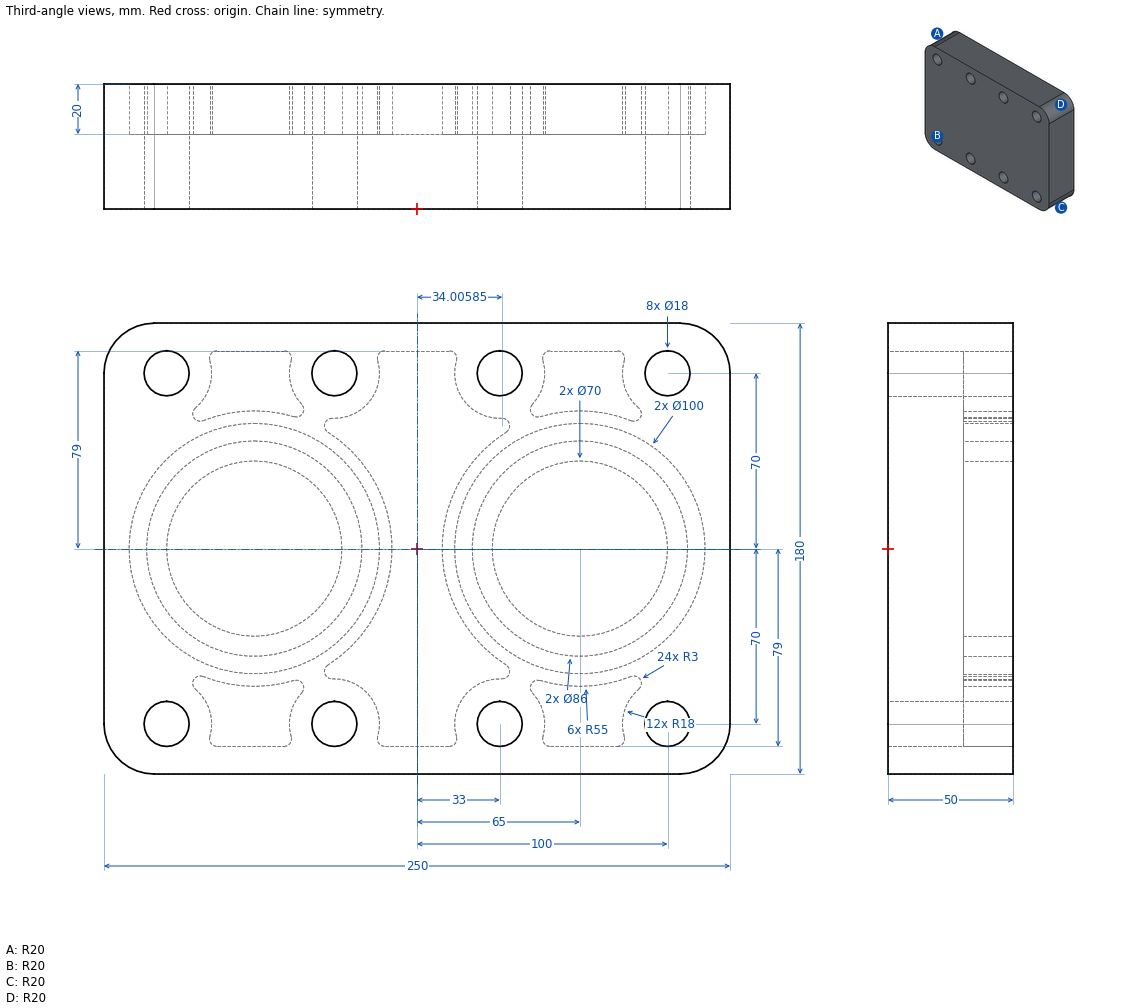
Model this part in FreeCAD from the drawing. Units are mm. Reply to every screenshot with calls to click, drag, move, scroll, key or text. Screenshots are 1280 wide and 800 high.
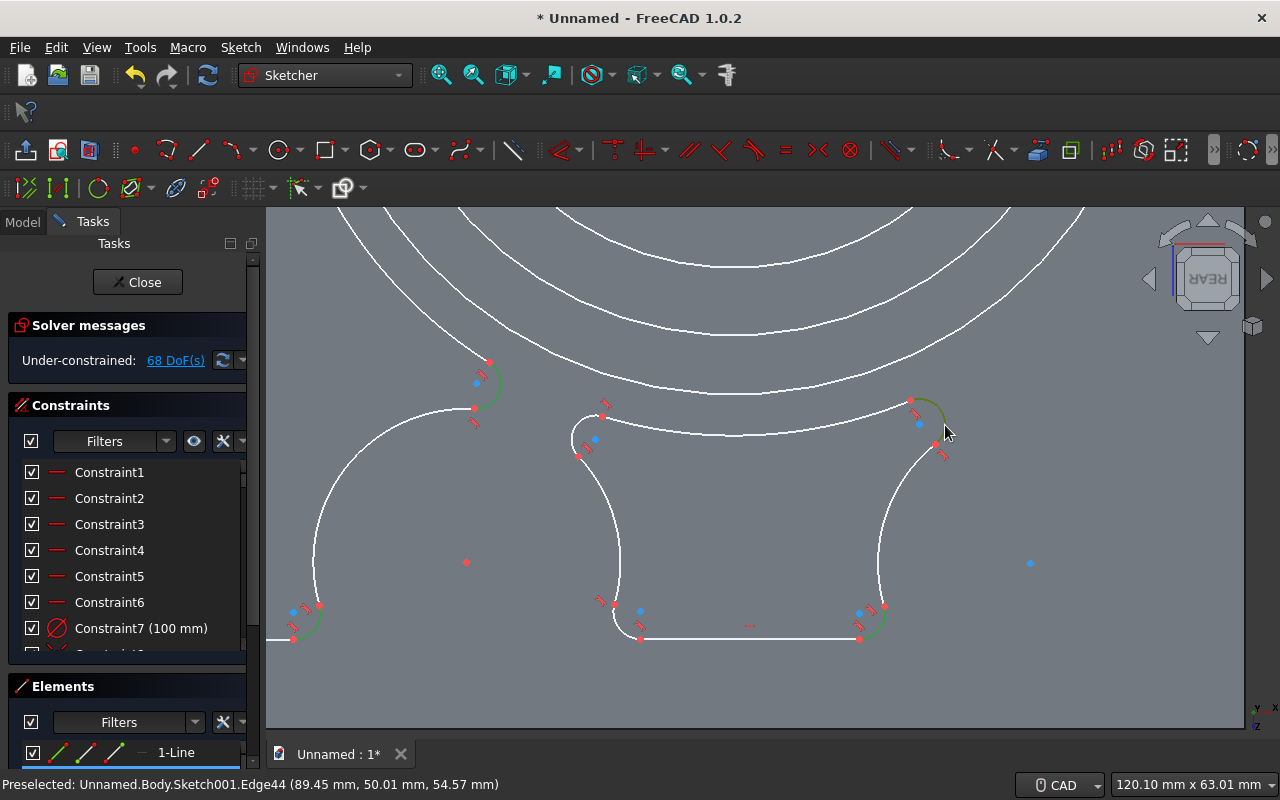
click(584, 418)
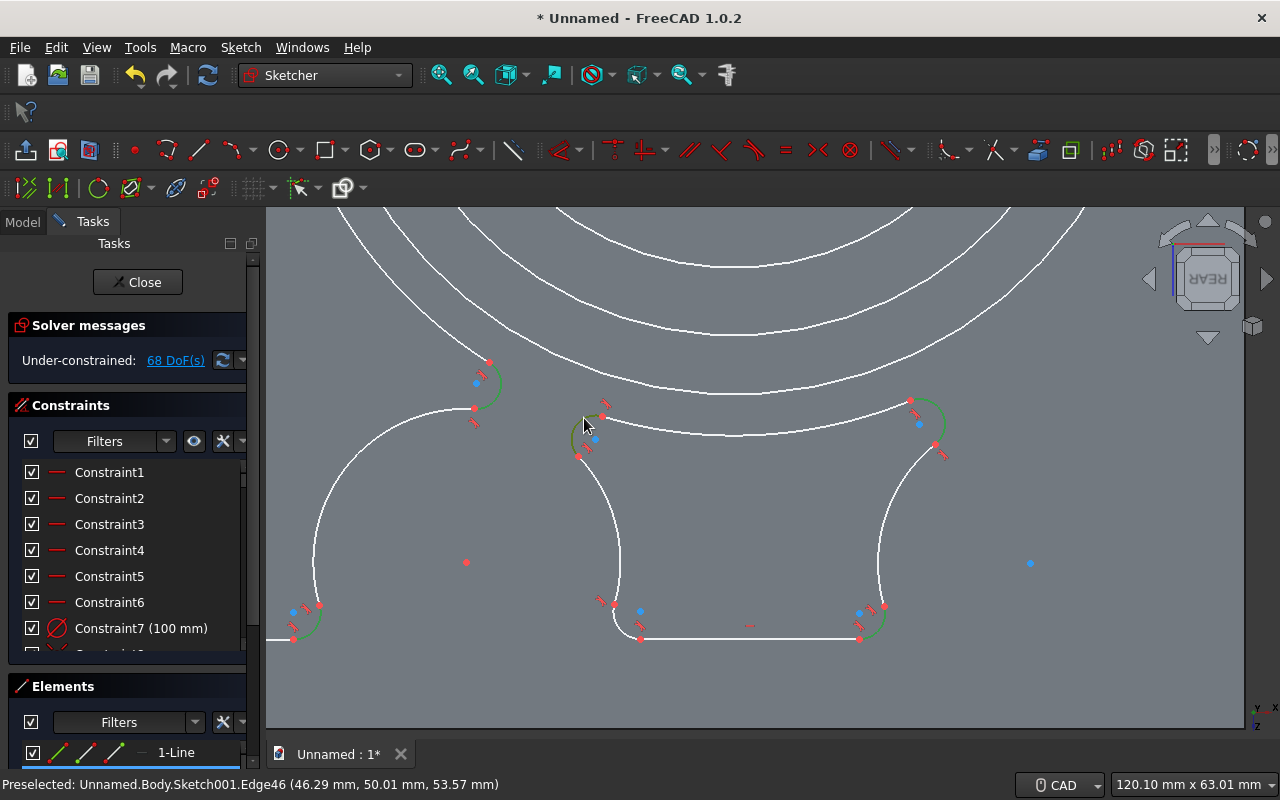
click(615, 619)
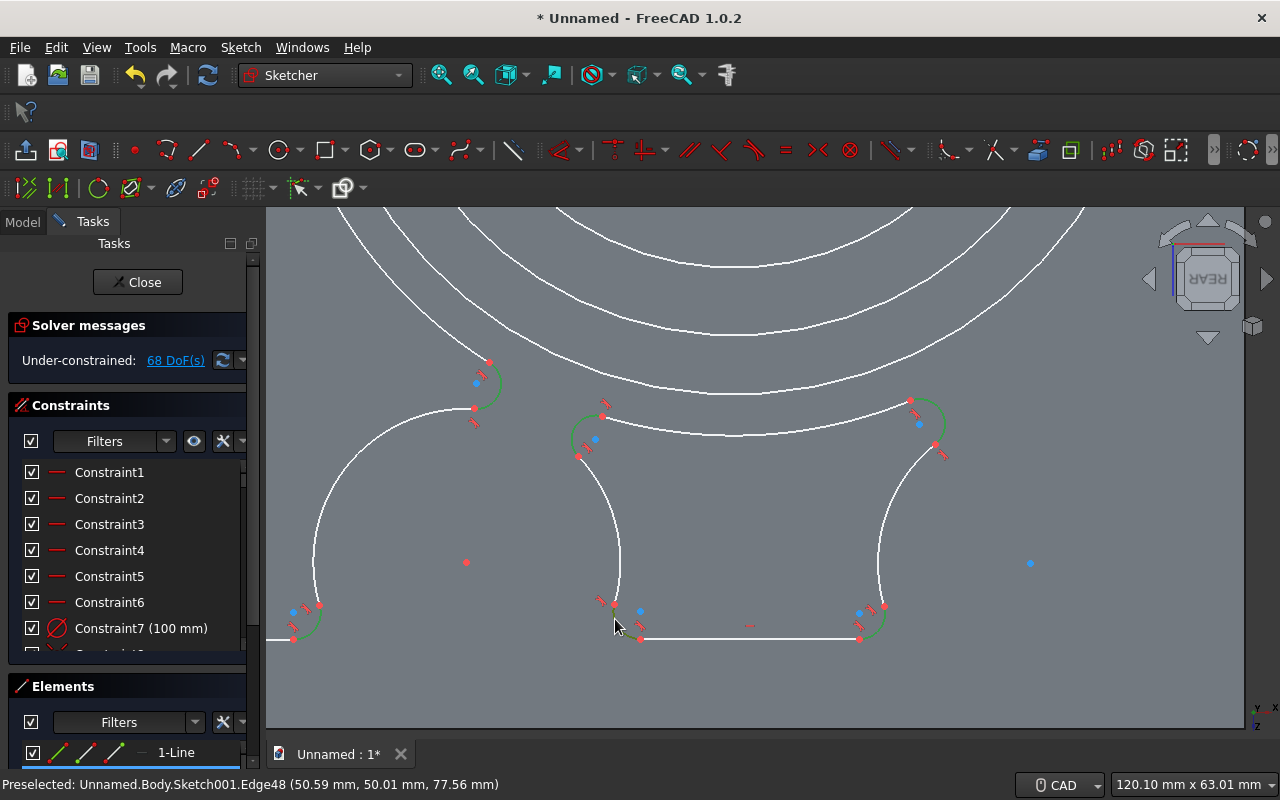
click(786, 150)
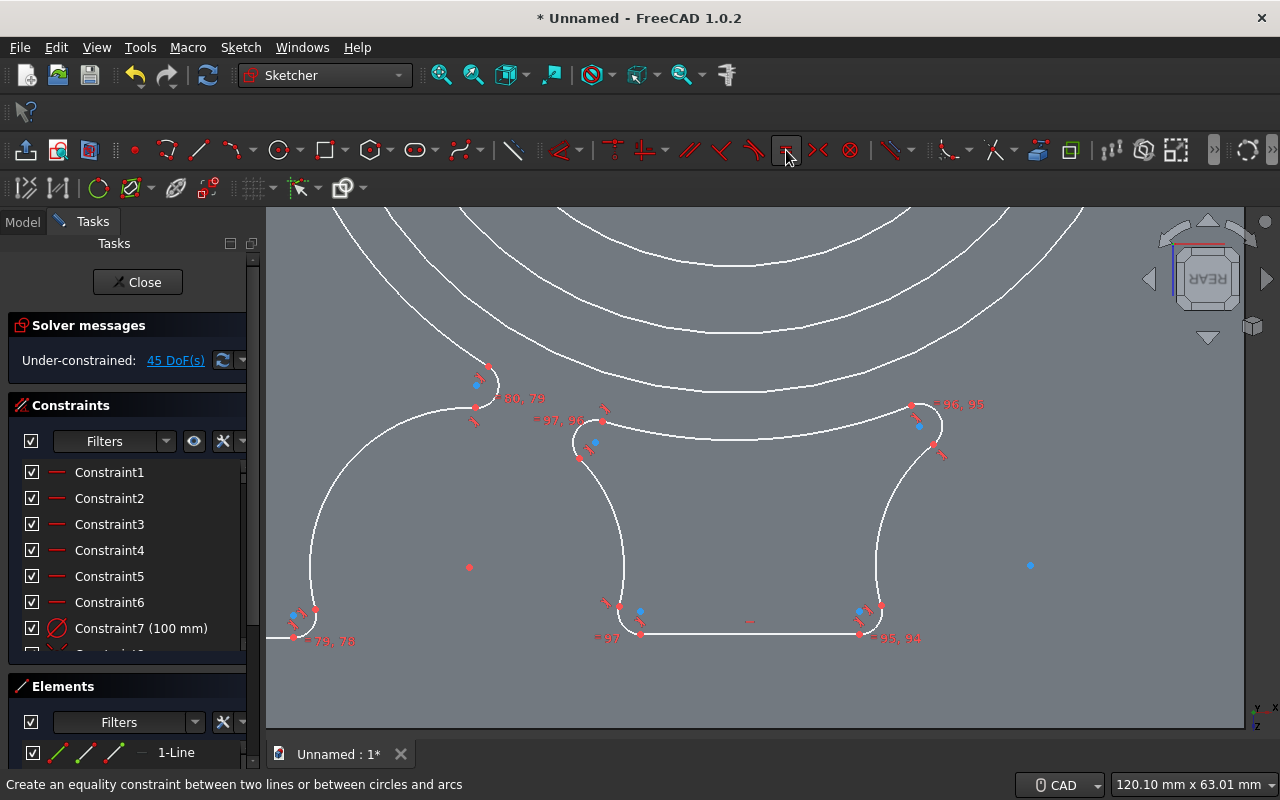
scroll(873, 638, down, 7)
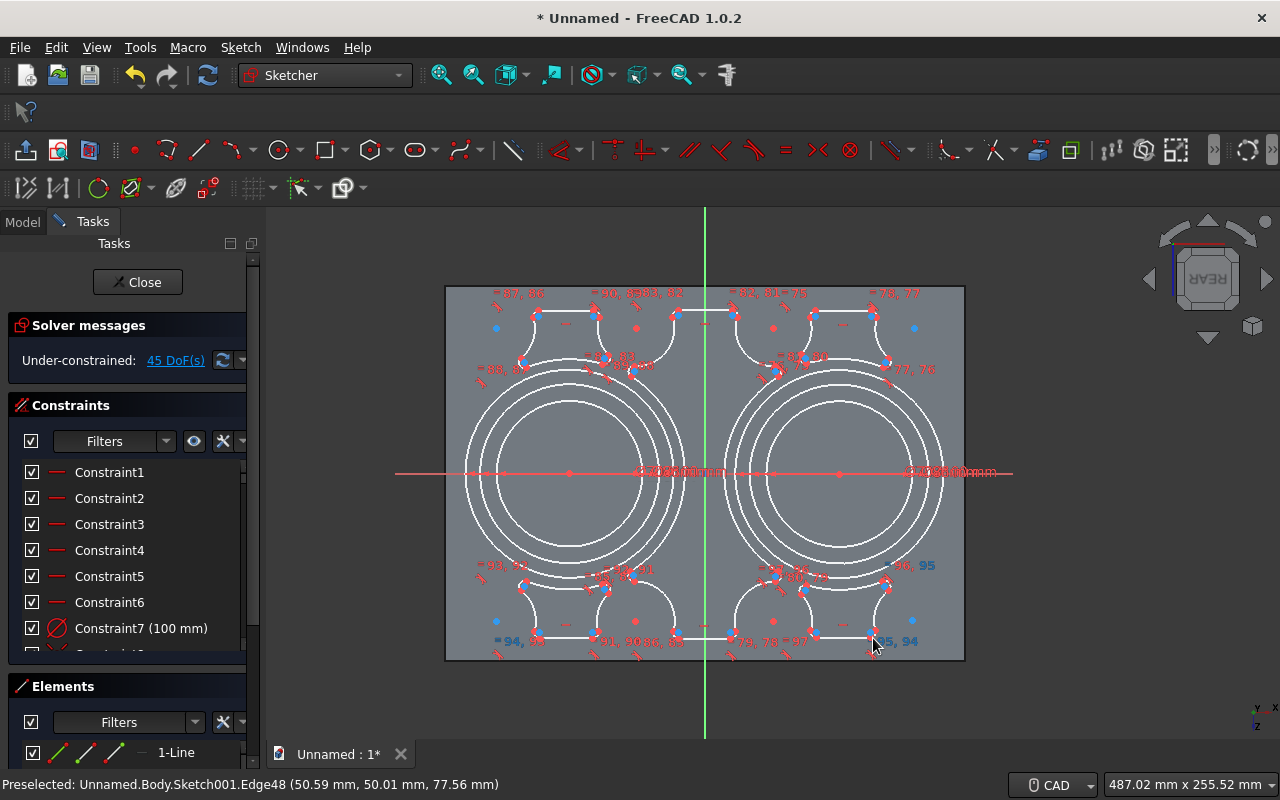
click(808, 345)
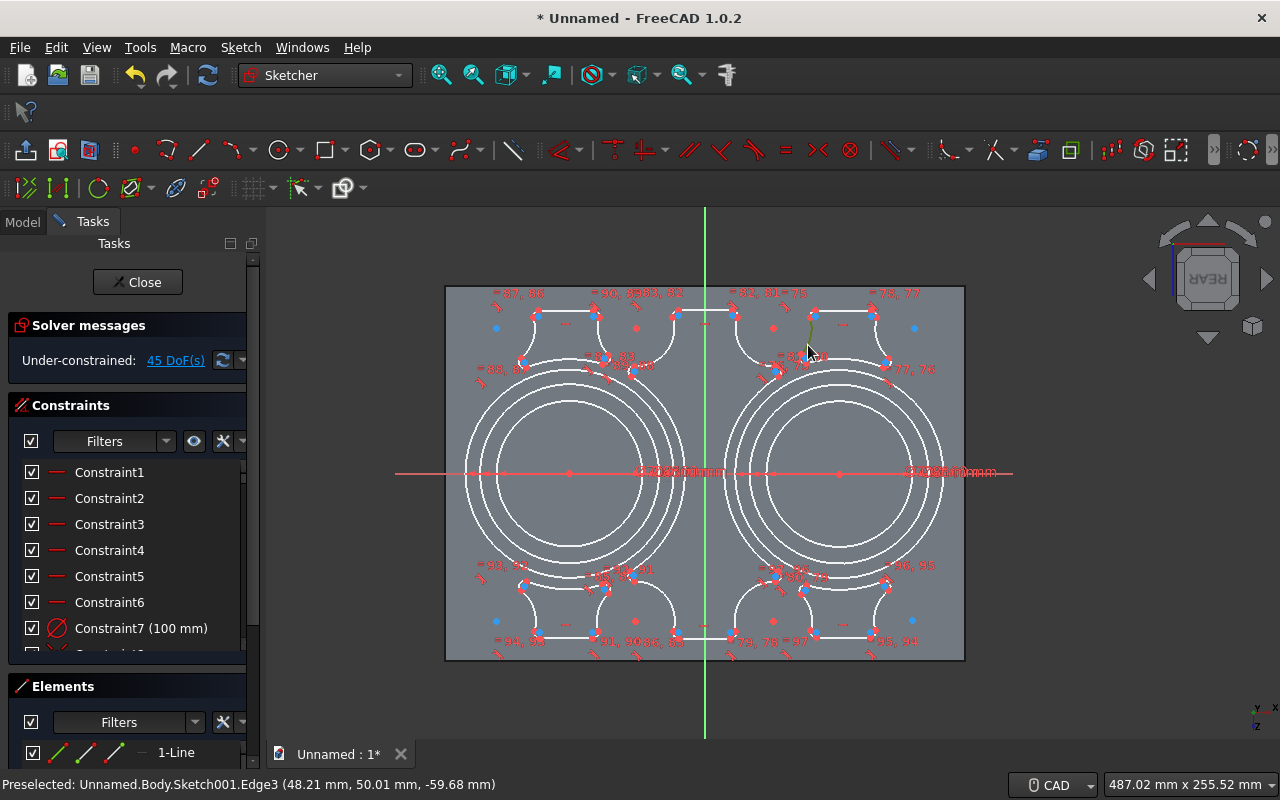
click(875, 331)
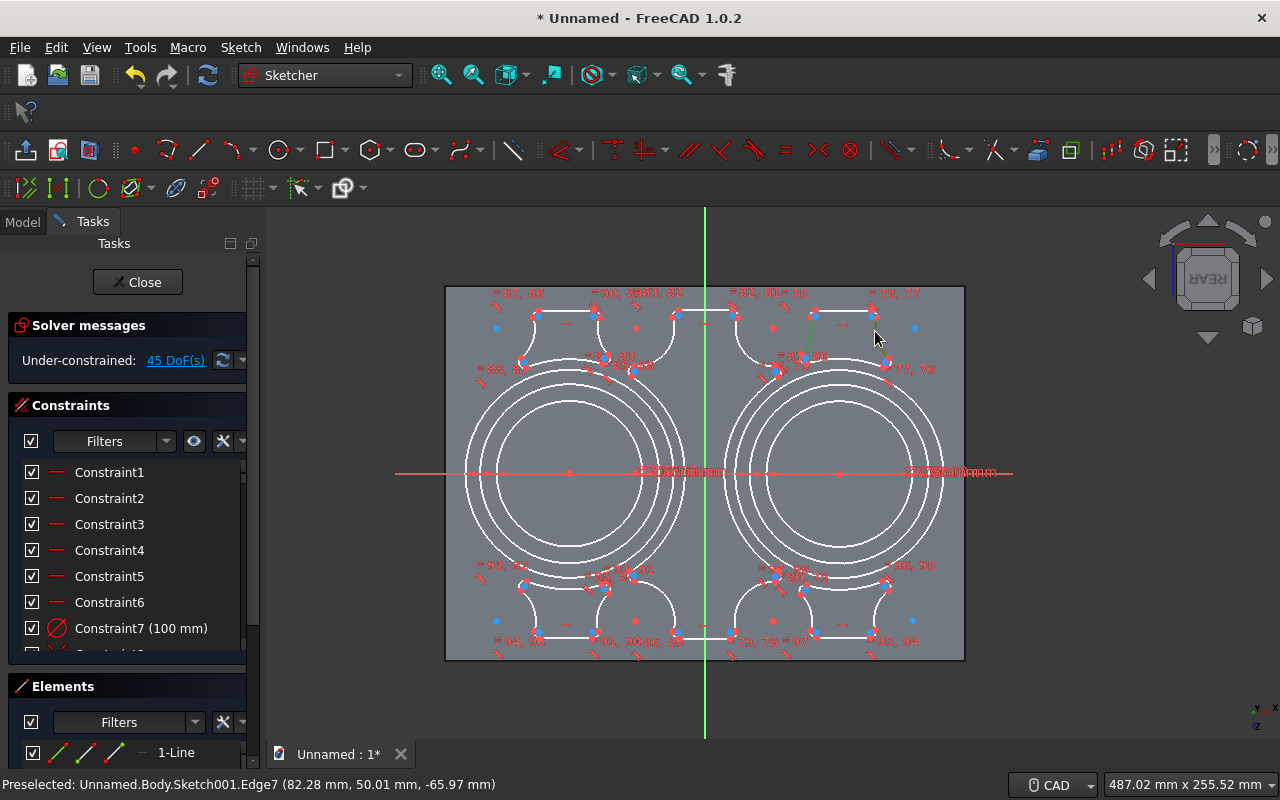
click(754, 587)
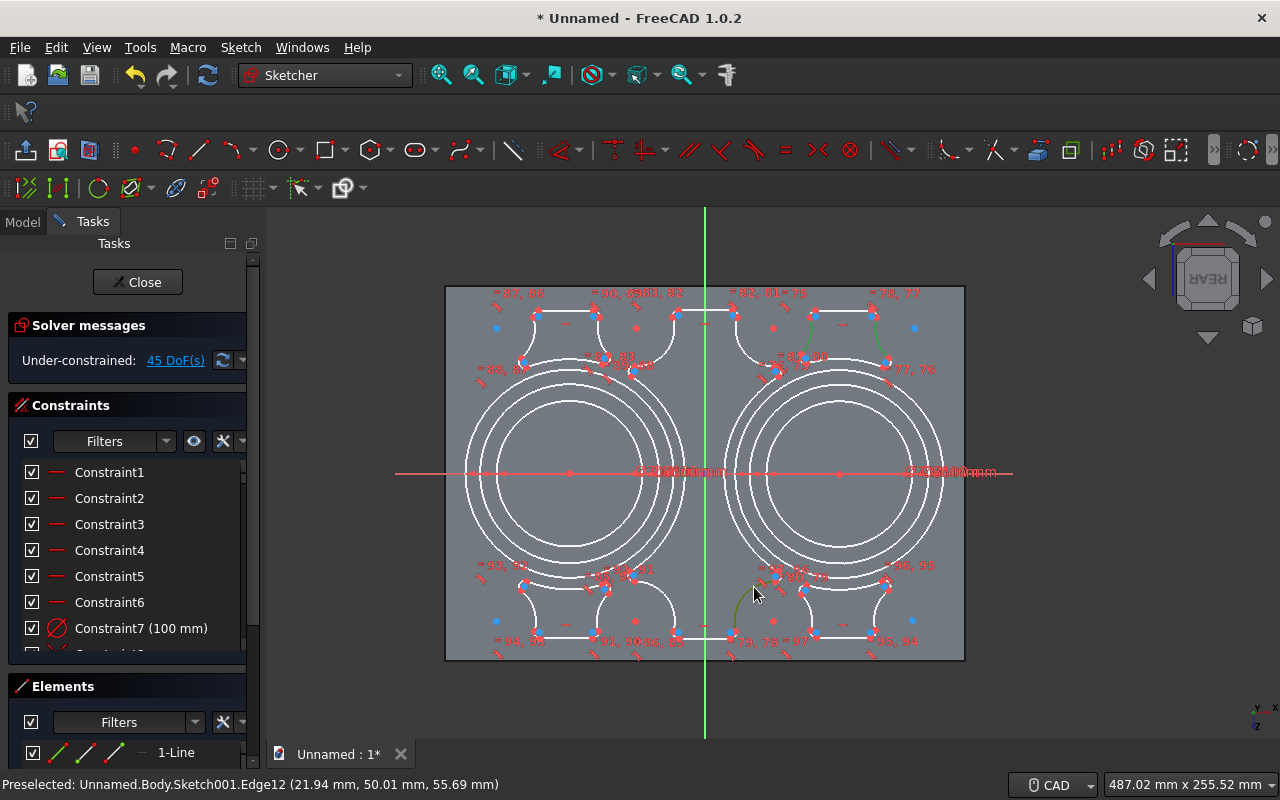
click(737, 339)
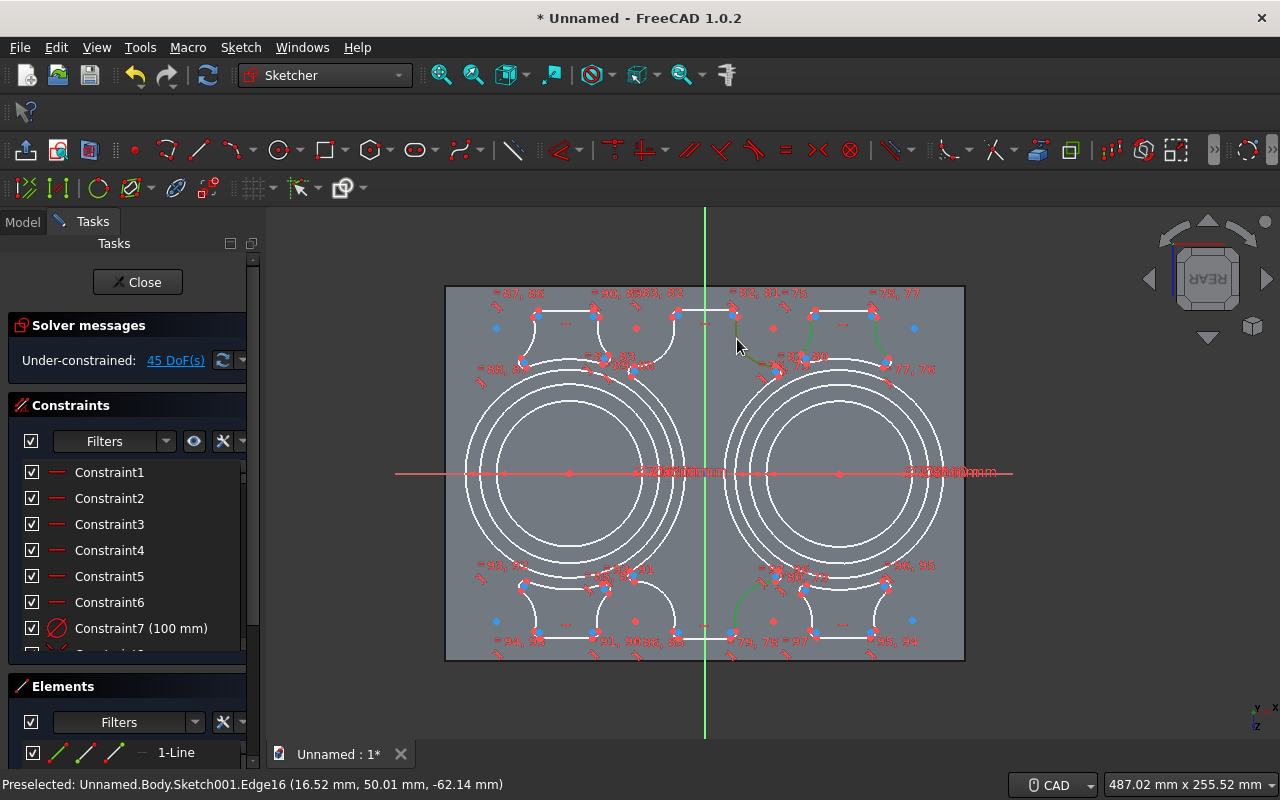
click(655, 361)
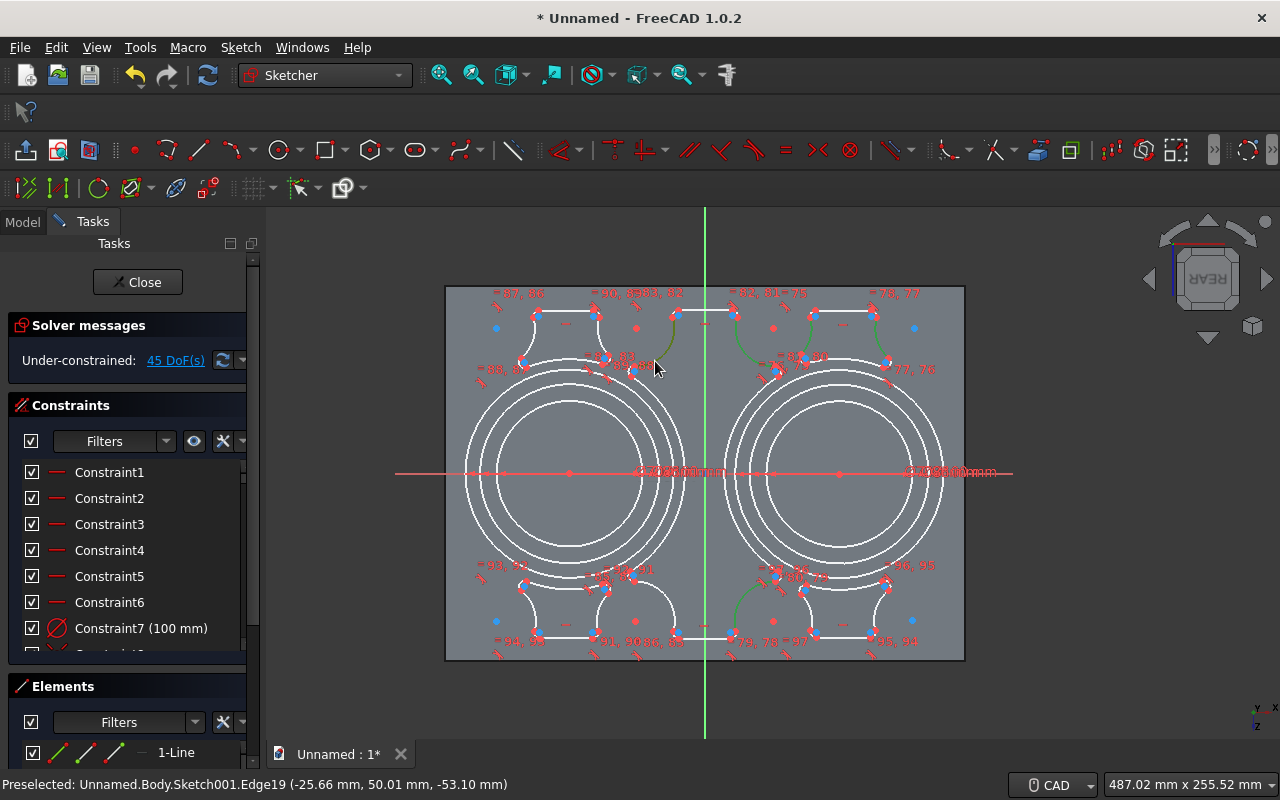
click(673, 610)